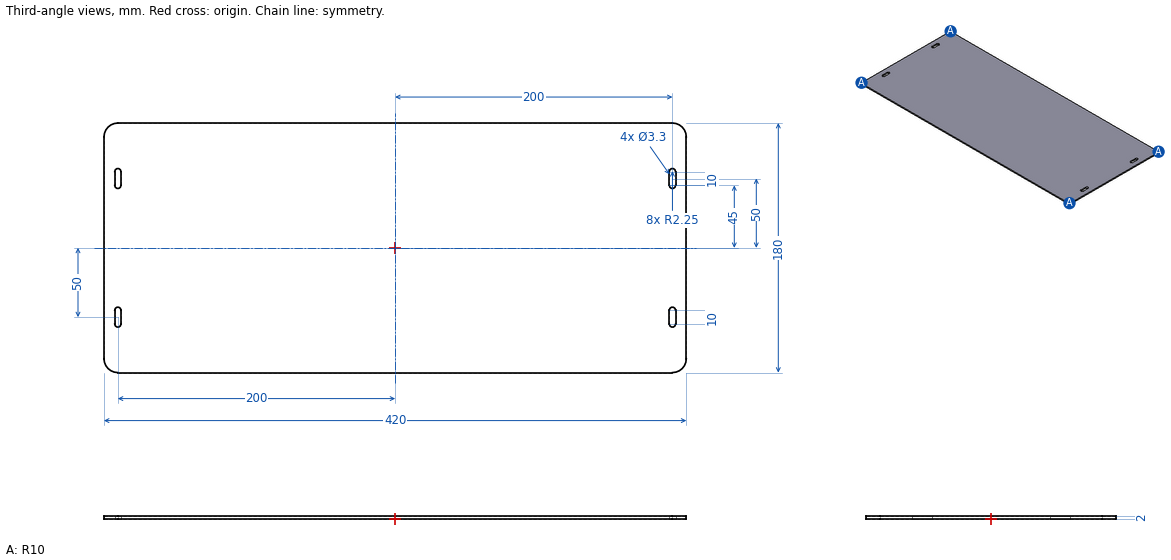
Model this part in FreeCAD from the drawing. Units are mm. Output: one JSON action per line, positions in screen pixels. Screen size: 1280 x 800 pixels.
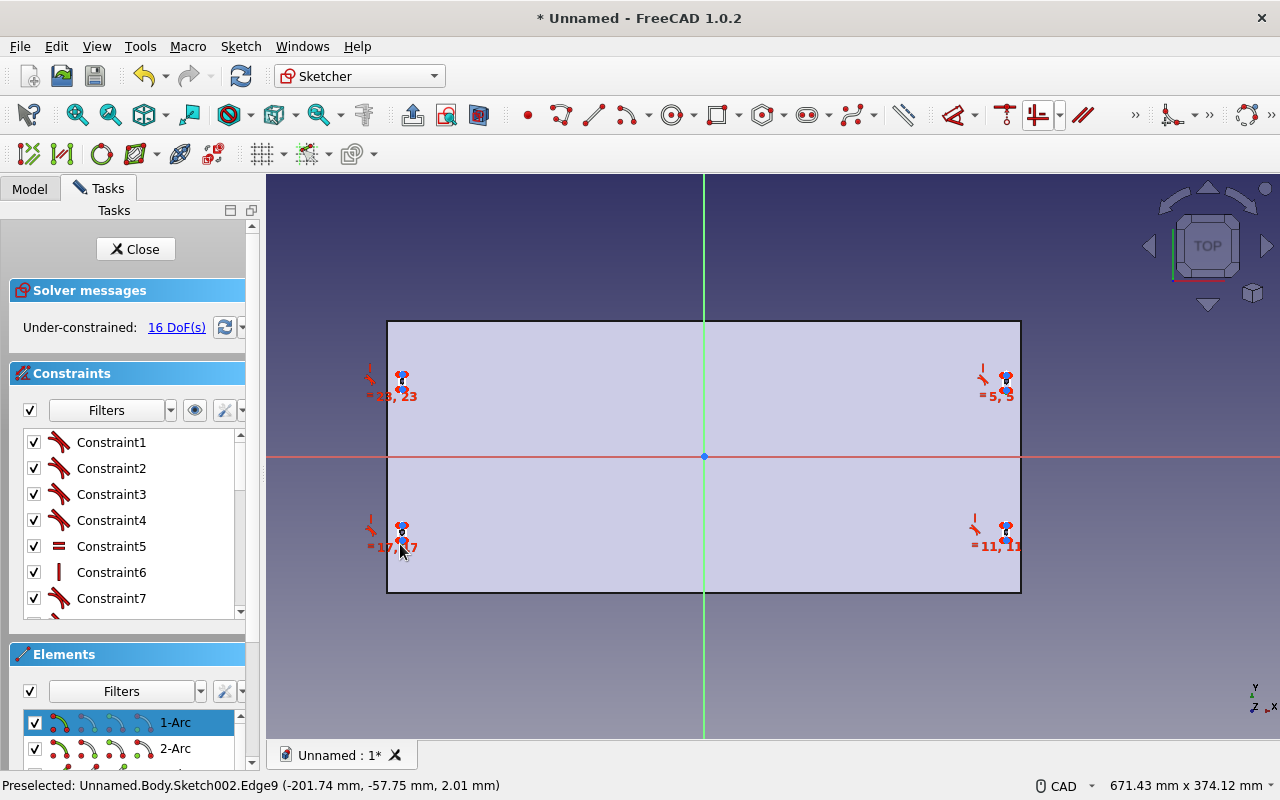
{"action": "scroll", "coordinate": [400, 393], "scroll_direction": "up", "scroll_amount": 8}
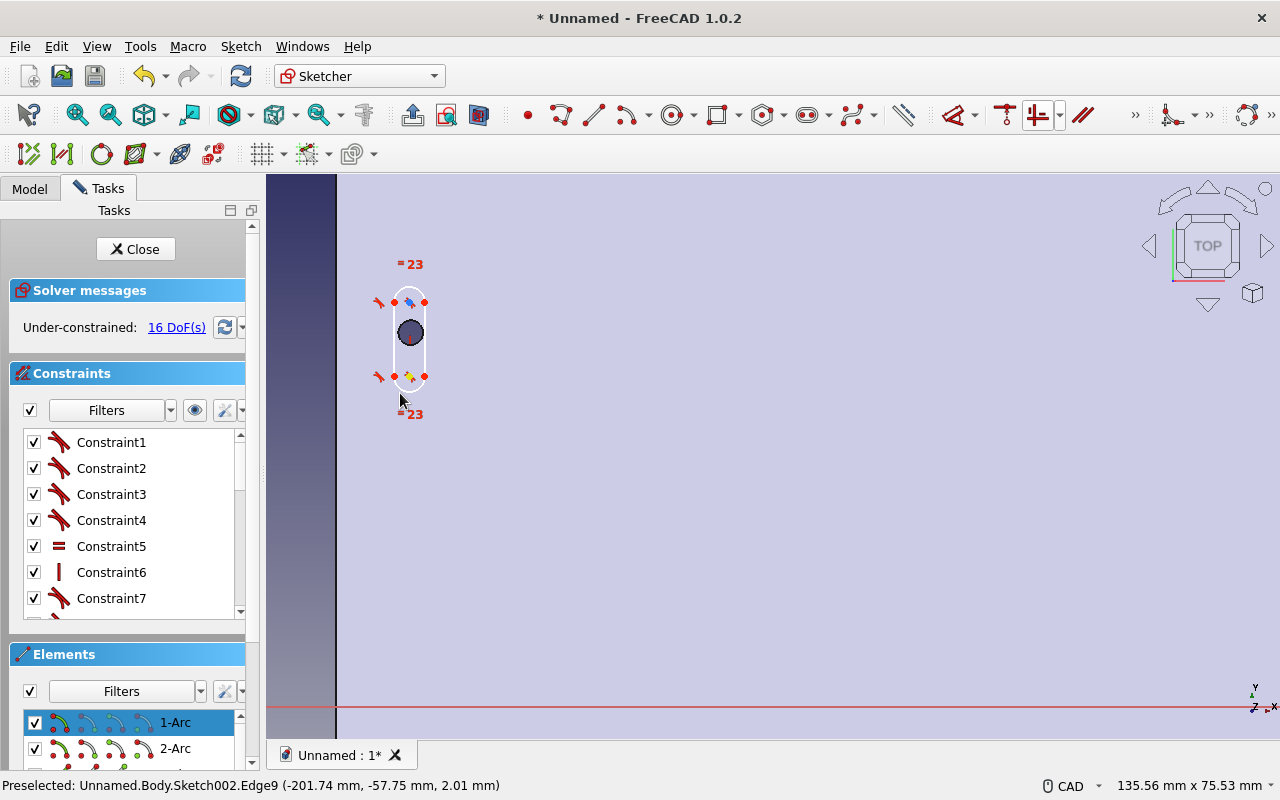
{"action": "left_click", "coordinate": [400, 389]}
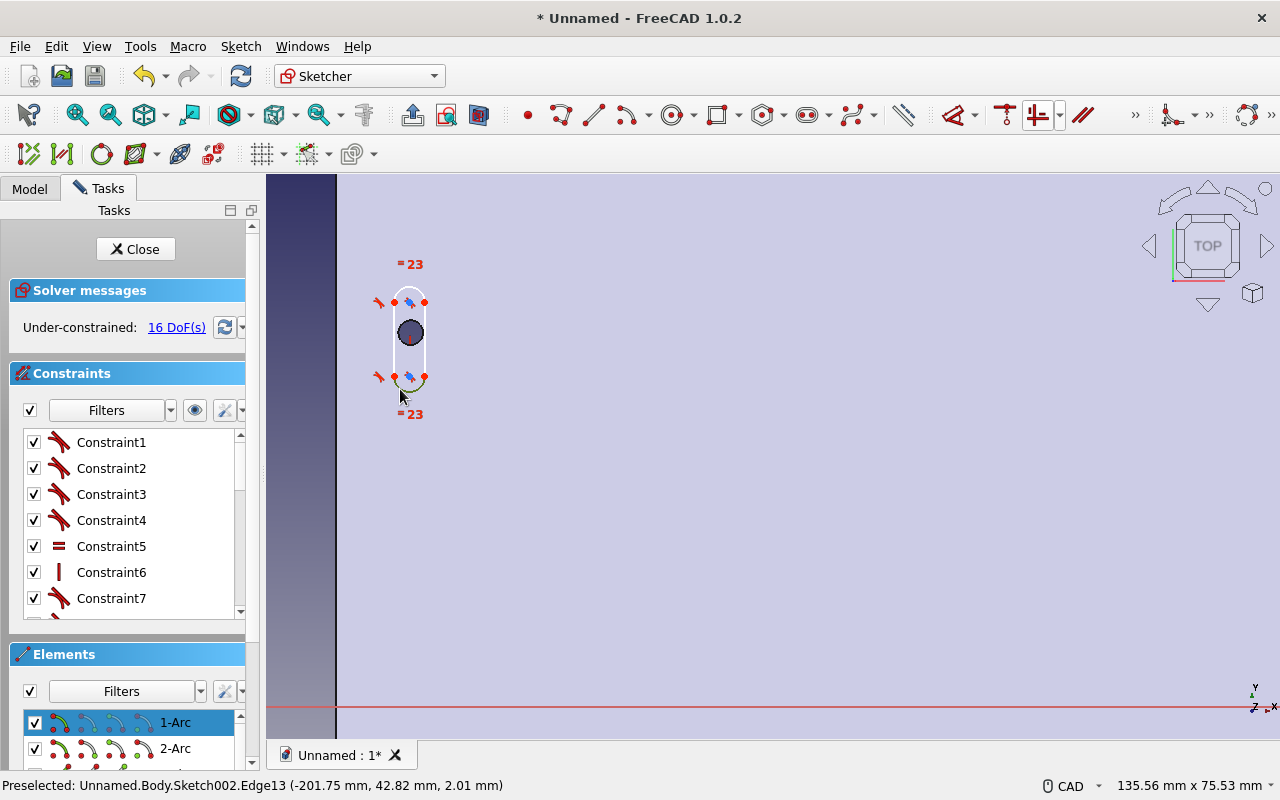
{"action": "key", "text": "e"}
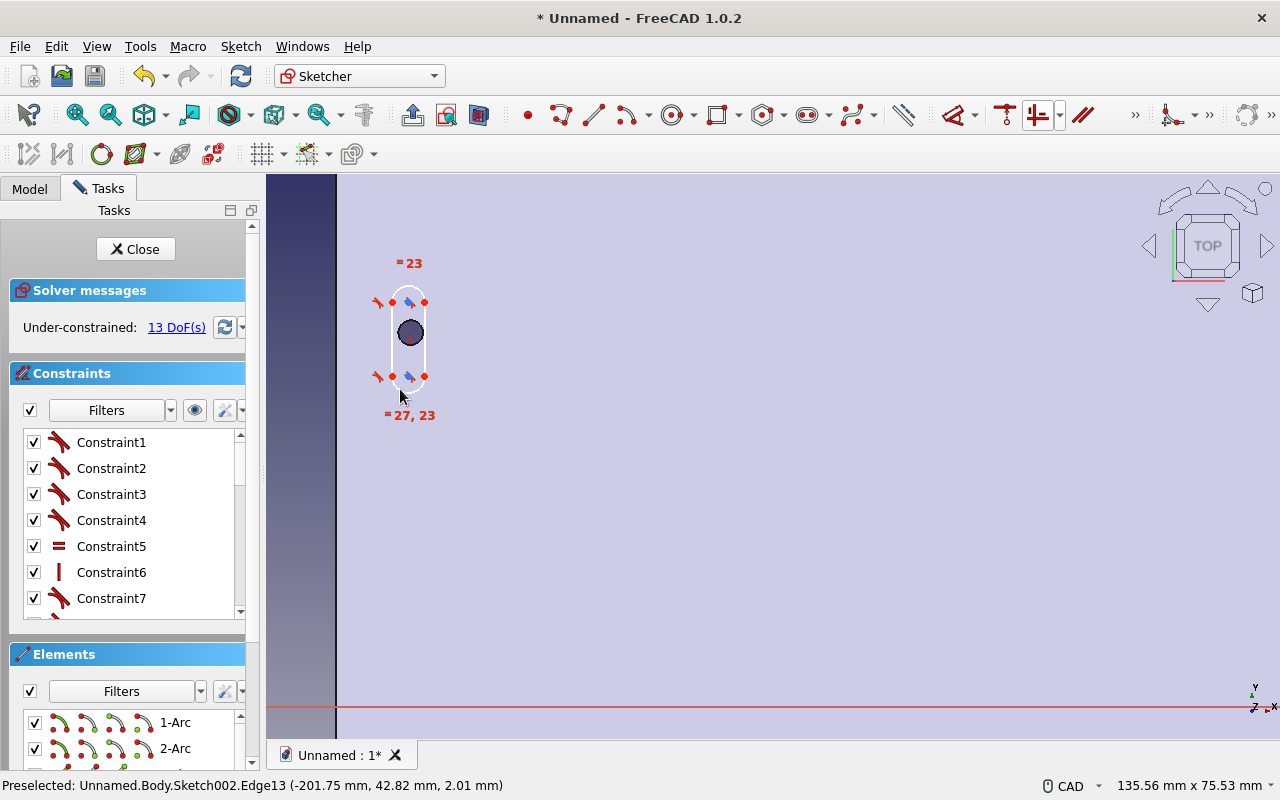
{"action": "scroll", "coordinate": [400, 393], "scroll_direction": "down", "scroll_amount": 8}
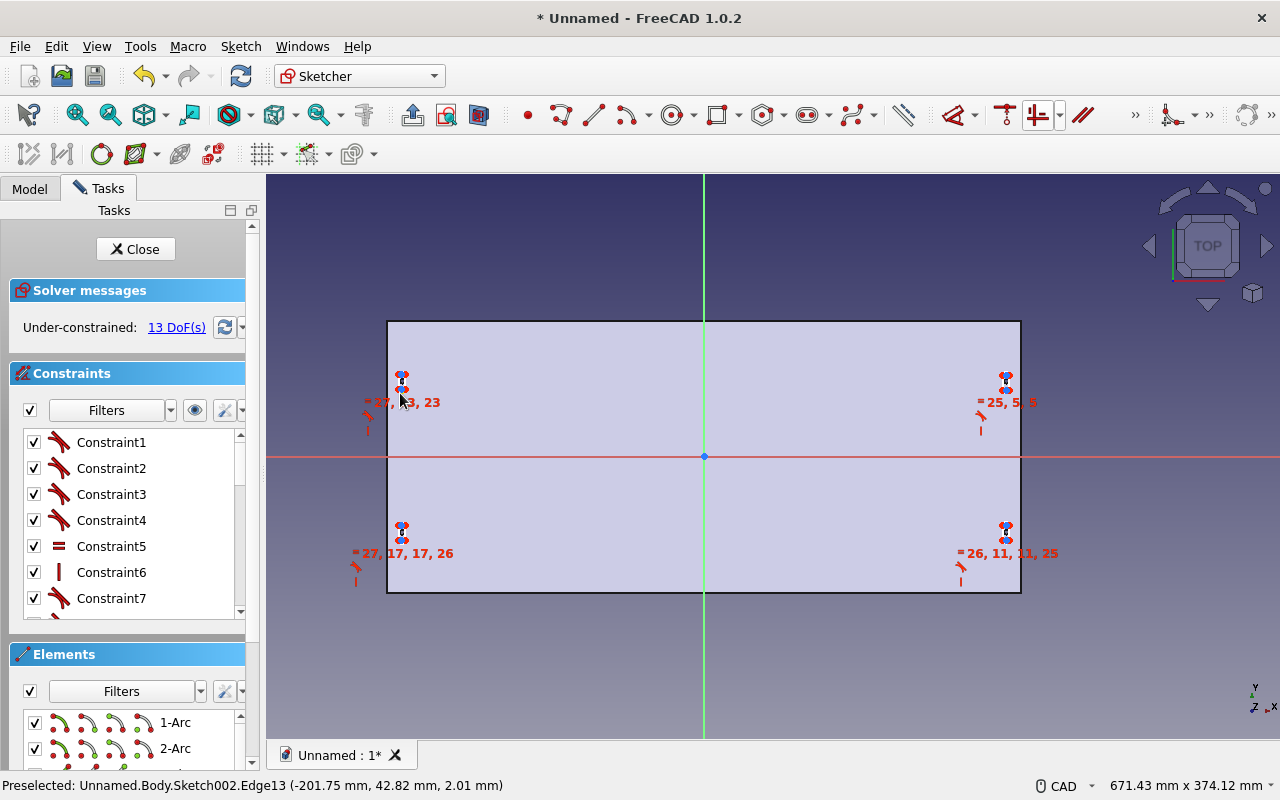
{"action": "scroll", "coordinate": [1006, 375], "scroll_direction": "up", "scroll_amount": 7}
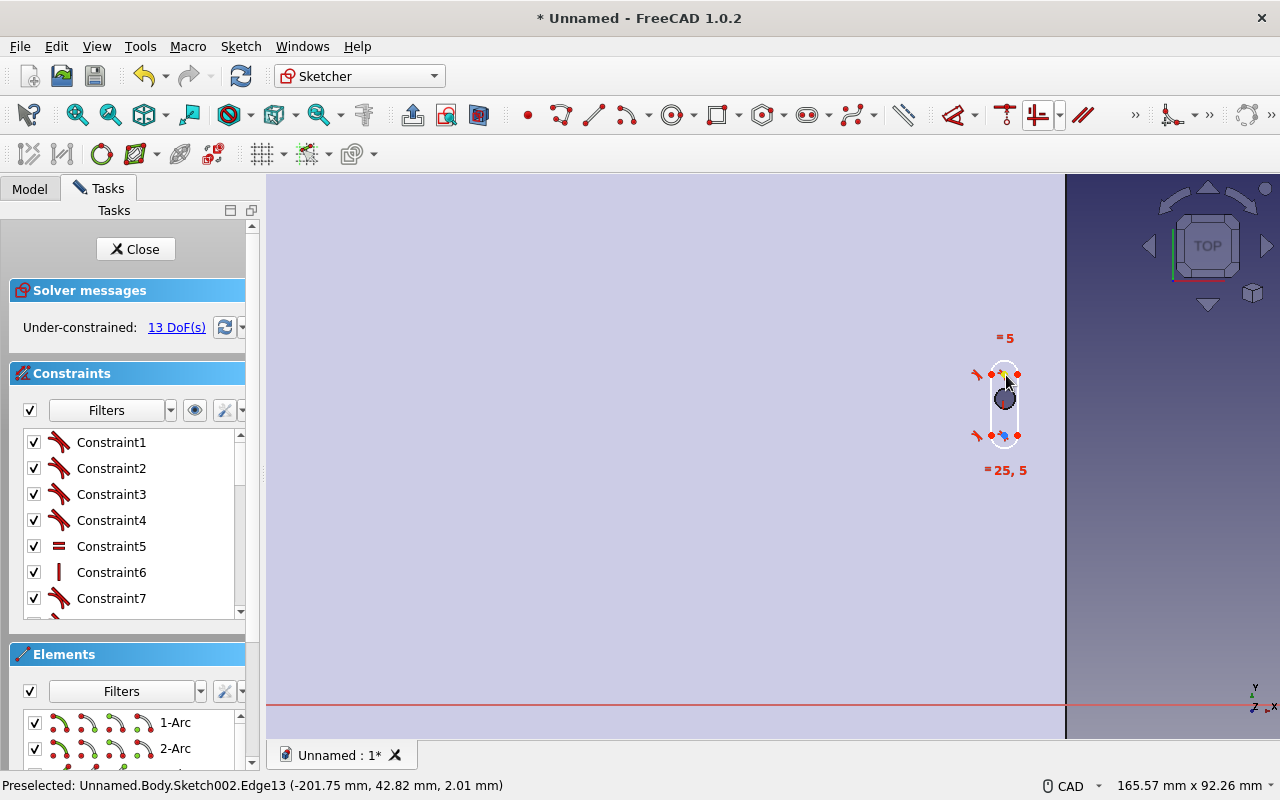
{"action": "left_click", "coordinate": [1005, 374]}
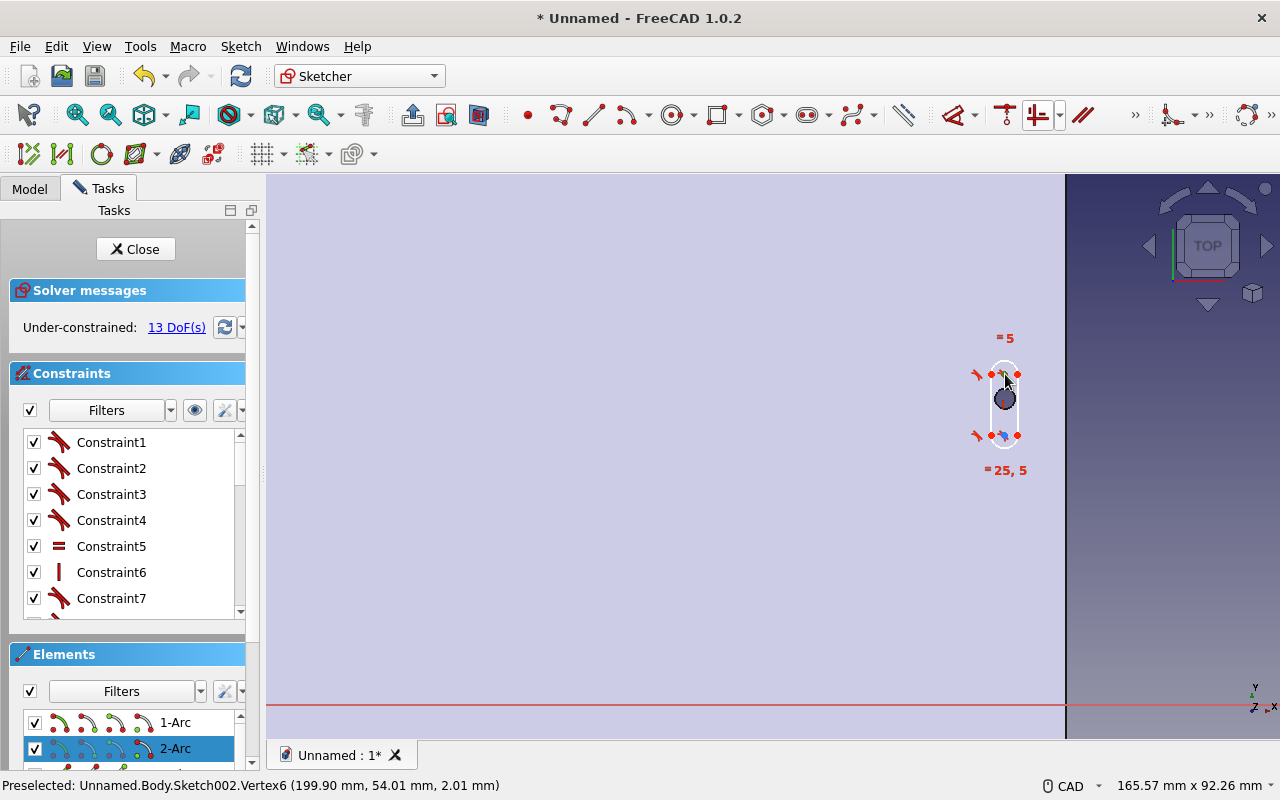
{"action": "scroll", "coordinate": [1007, 375], "scroll_direction": "down", "scroll_amount": 7}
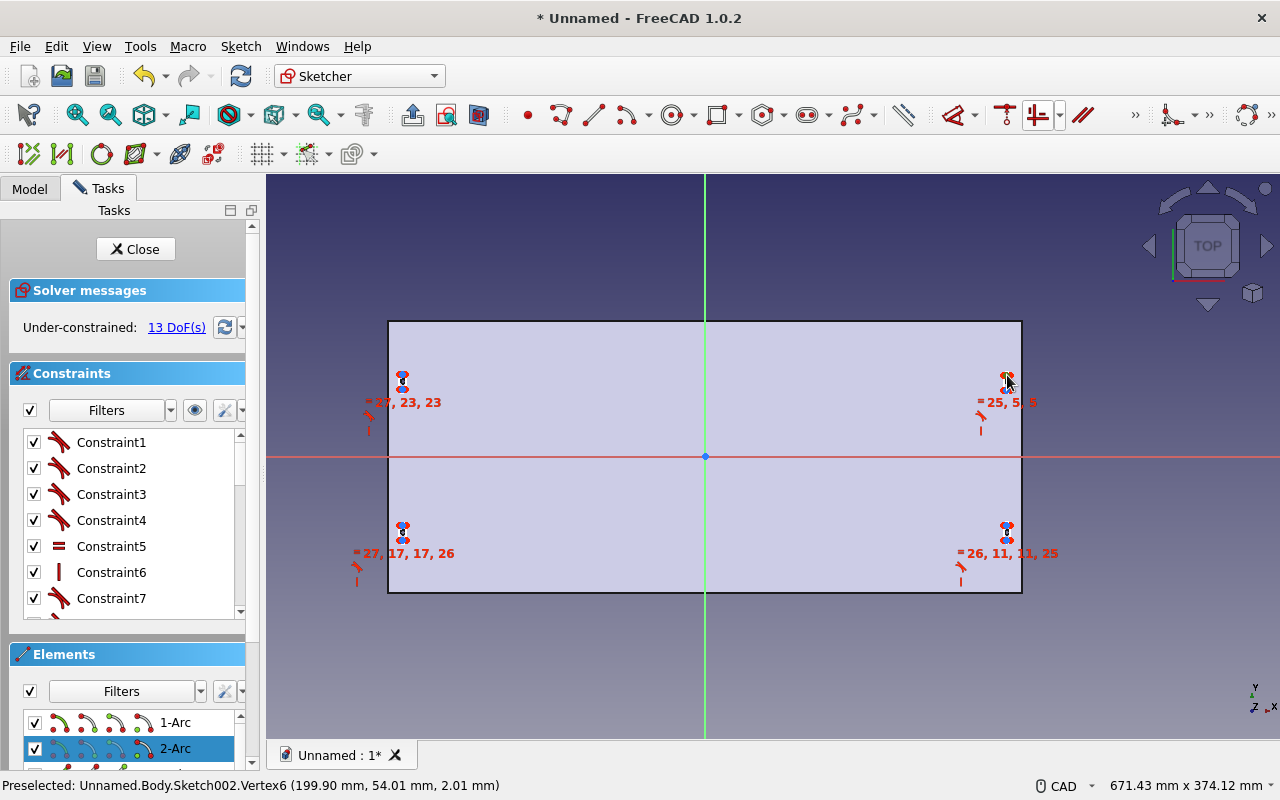
{"action": "scroll", "coordinate": [1007, 540], "scroll_direction": "up", "scroll_amount": 7}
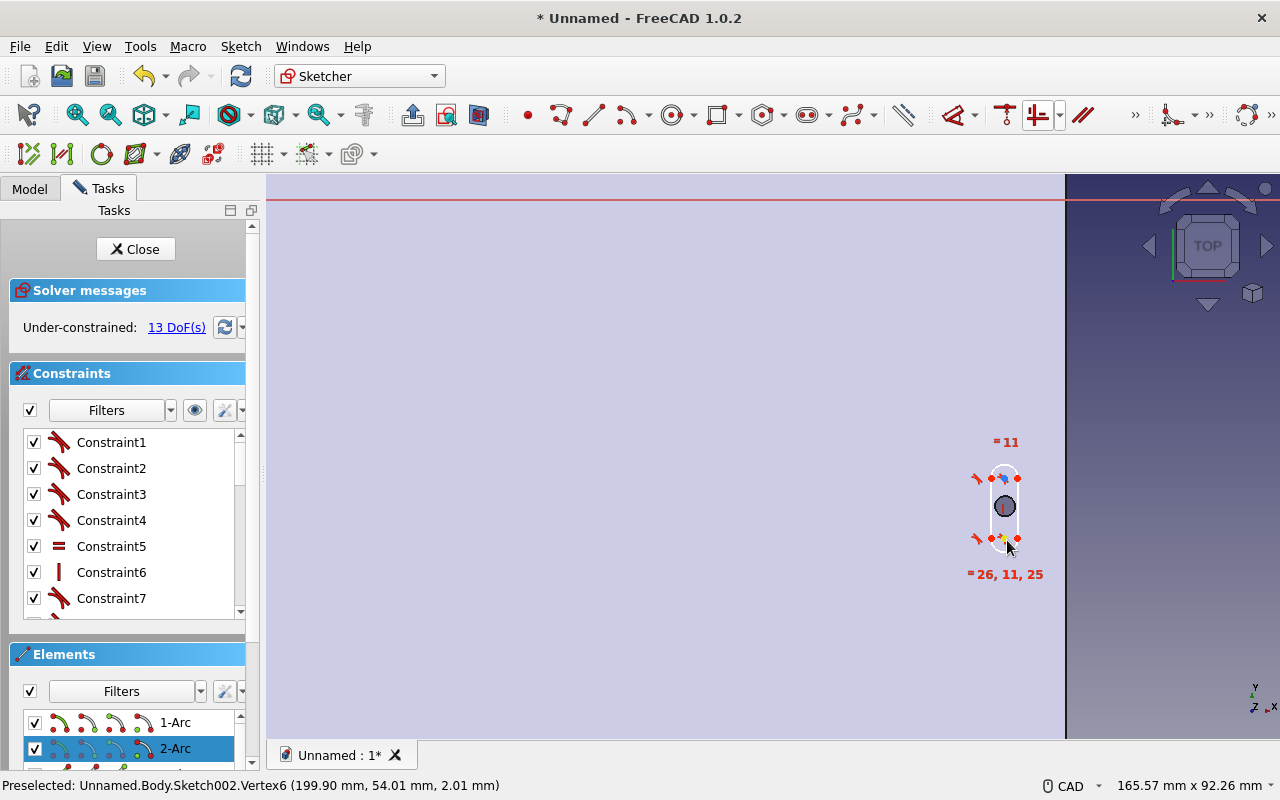
{"action": "left_click", "coordinate": [1004, 539]}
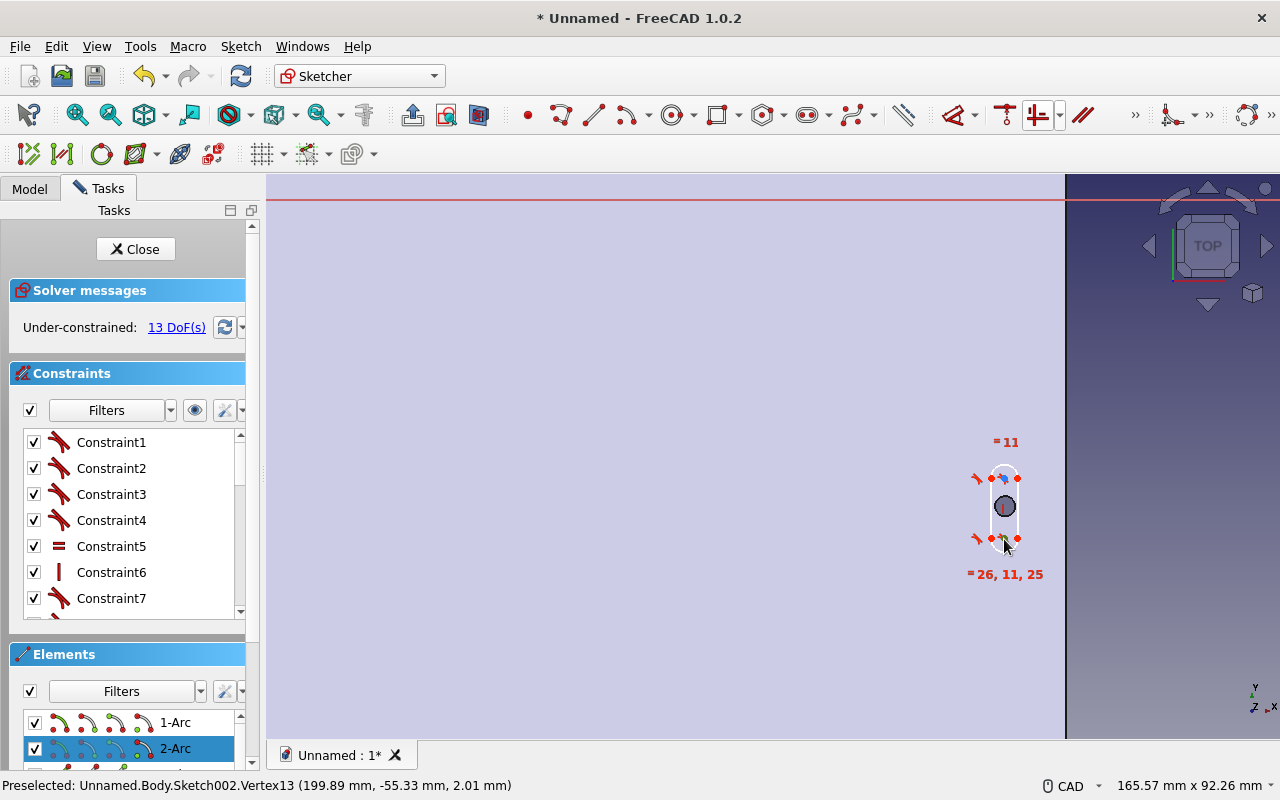
{"action": "scroll", "coordinate": [1007, 540], "scroll_direction": "down", "scroll_amount": 7}